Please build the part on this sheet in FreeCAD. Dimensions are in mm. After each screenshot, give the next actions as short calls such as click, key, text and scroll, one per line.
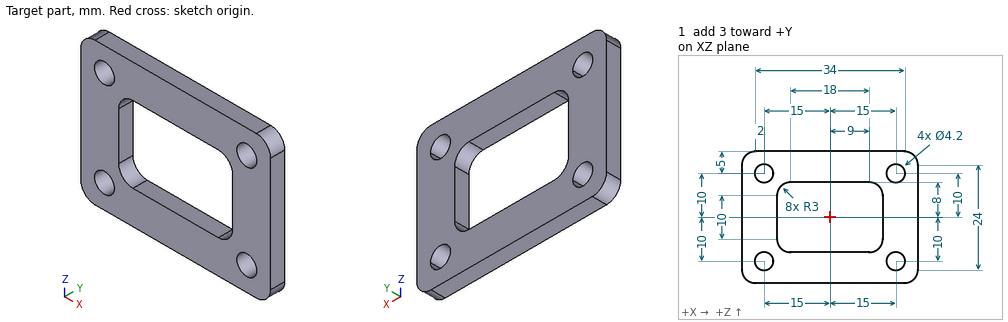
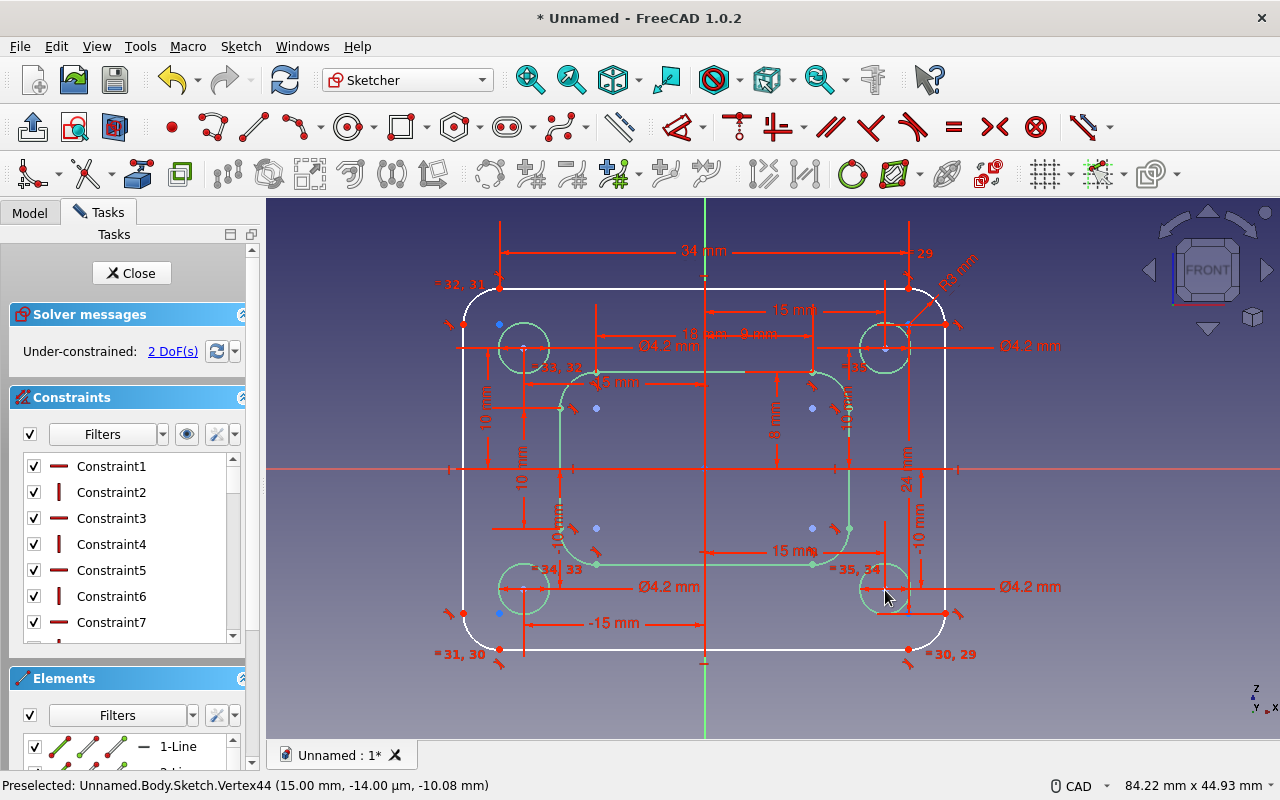
scroll(500, 289, up, 3)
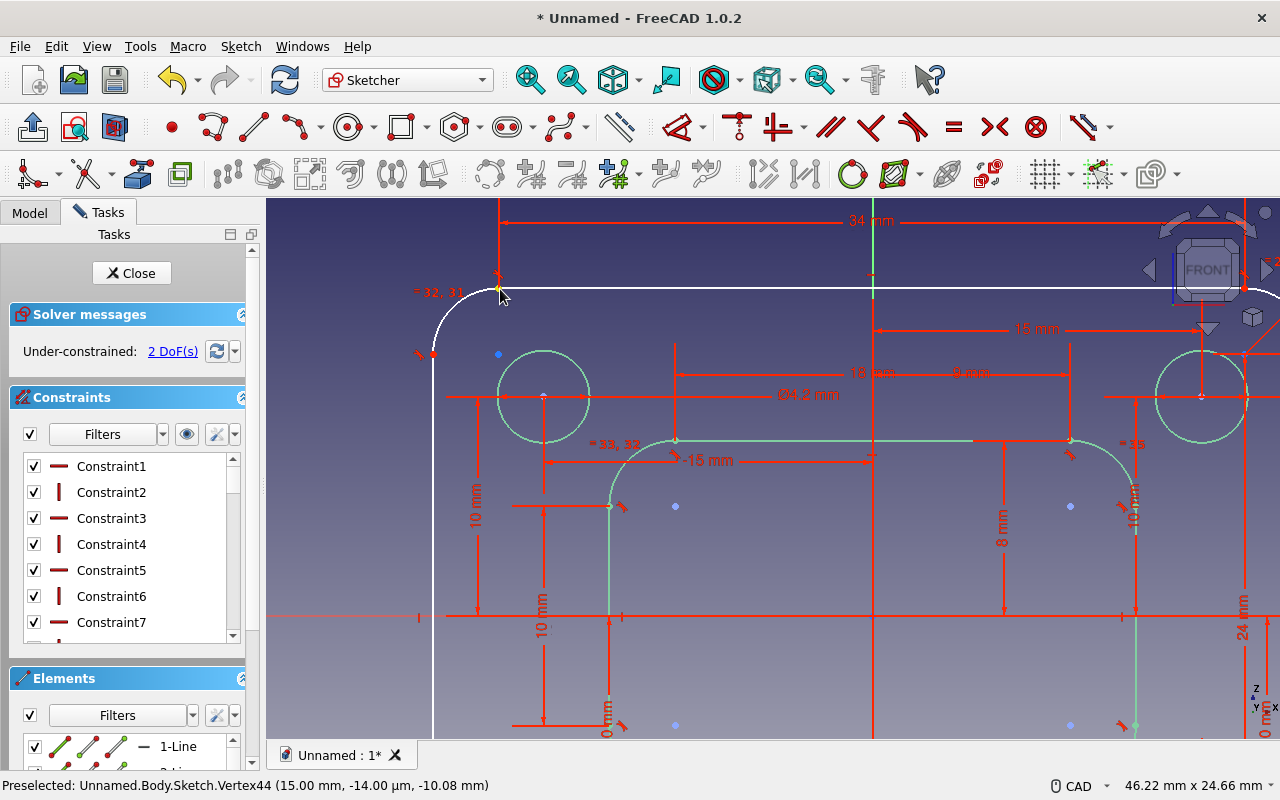
click(499, 288)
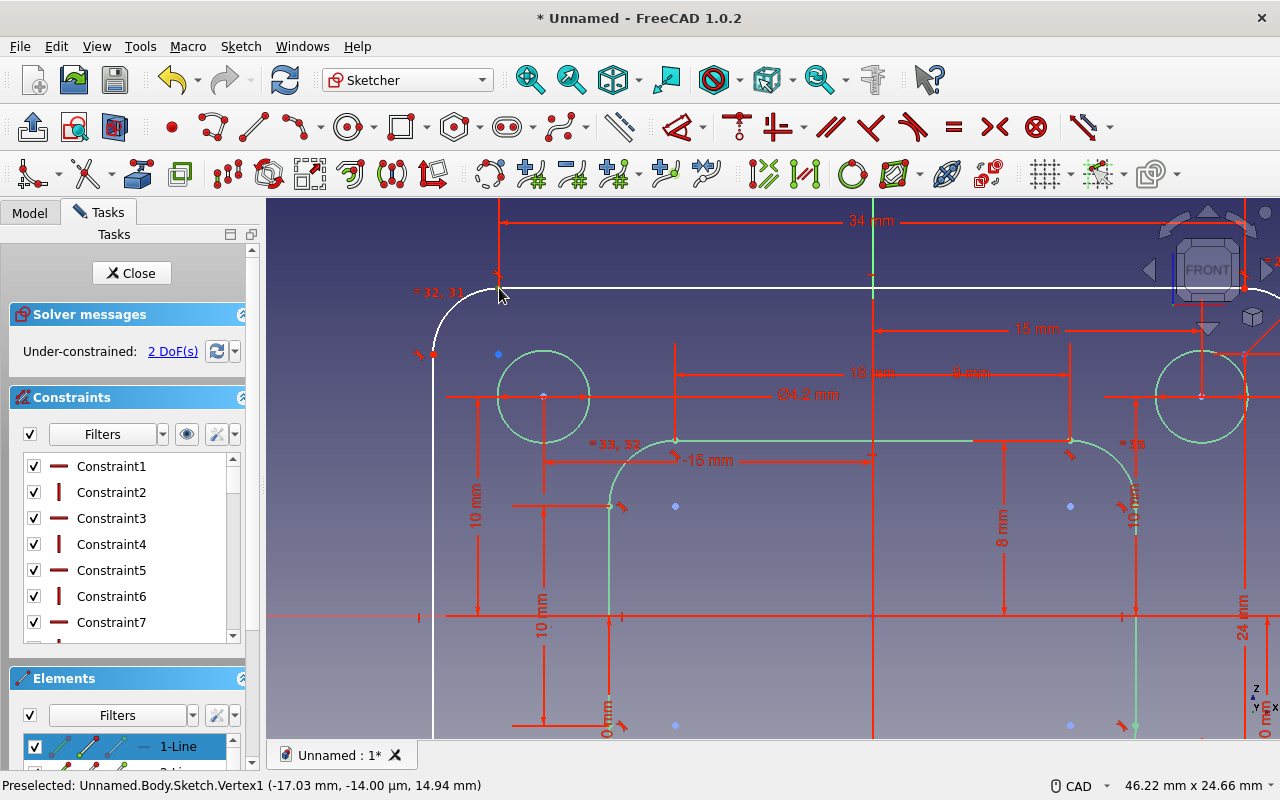
click(544, 397)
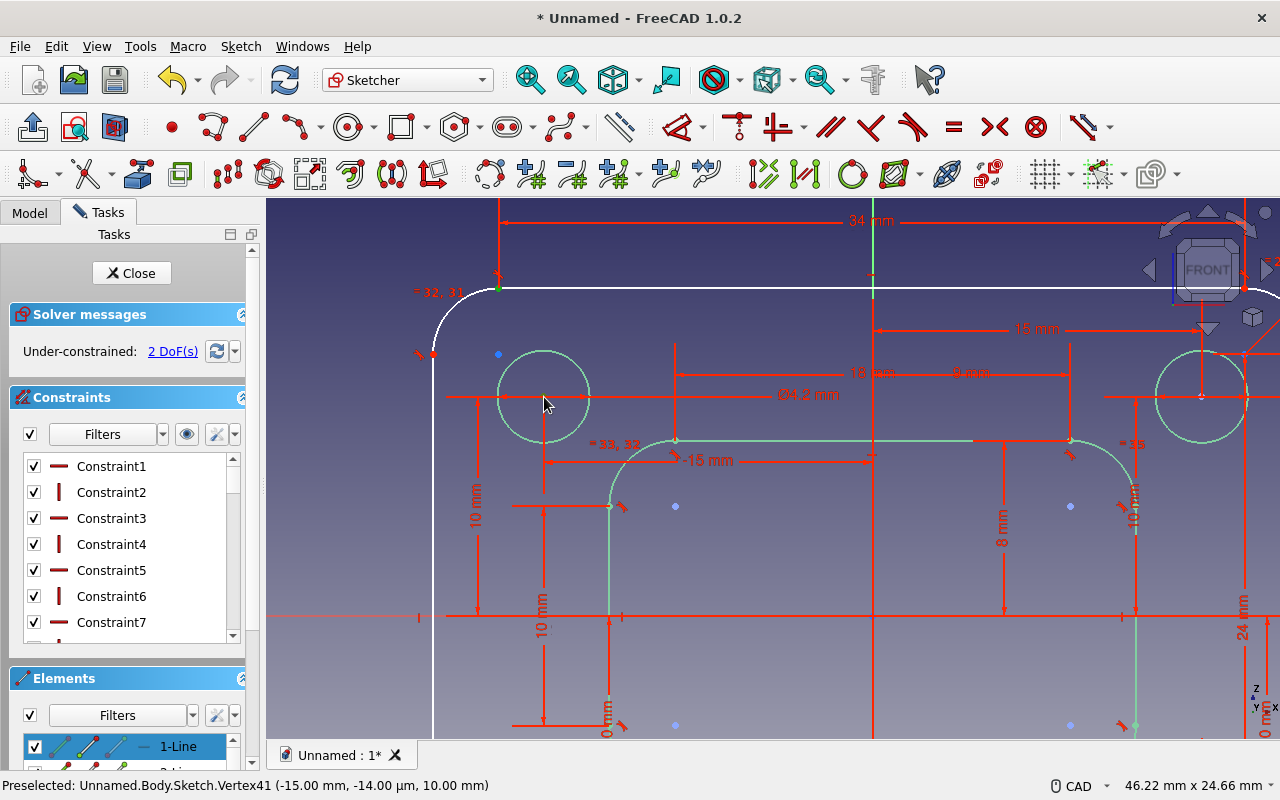
key(l)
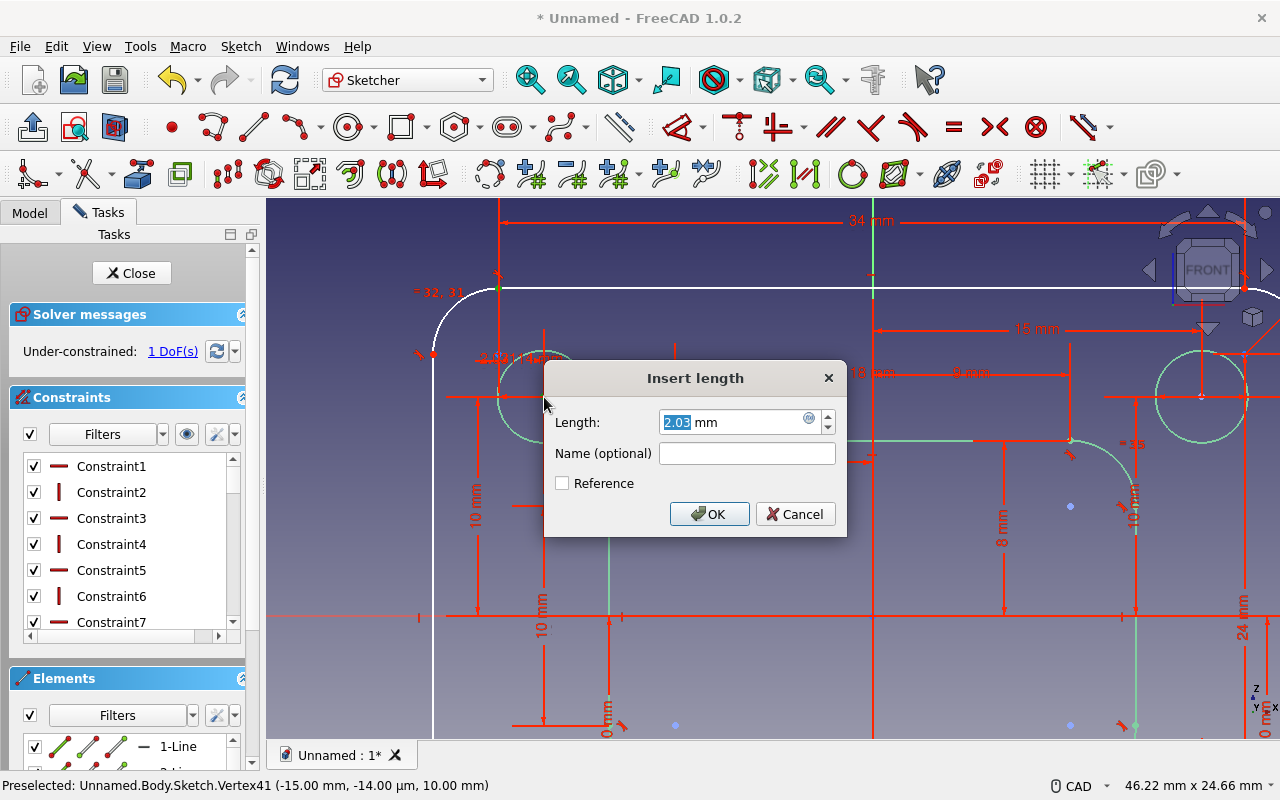
text(2)
key(Return)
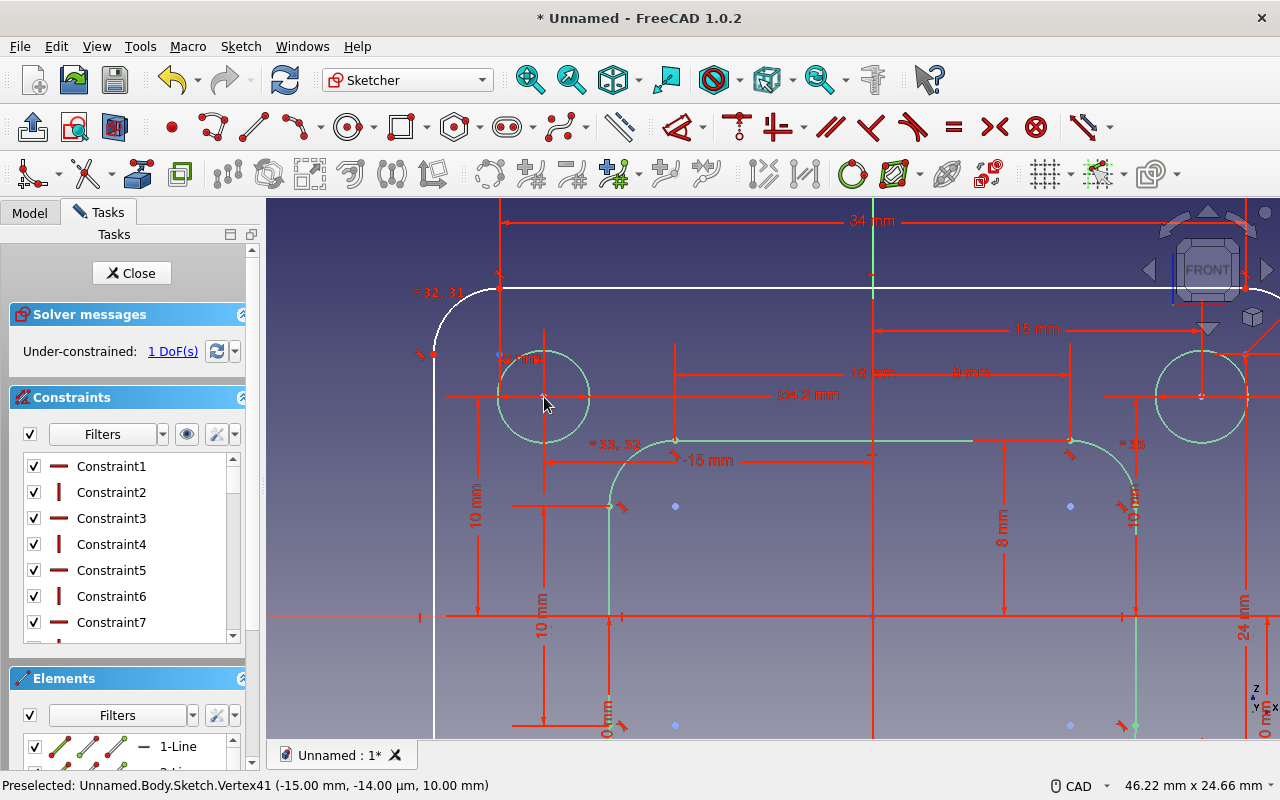
click(500, 288)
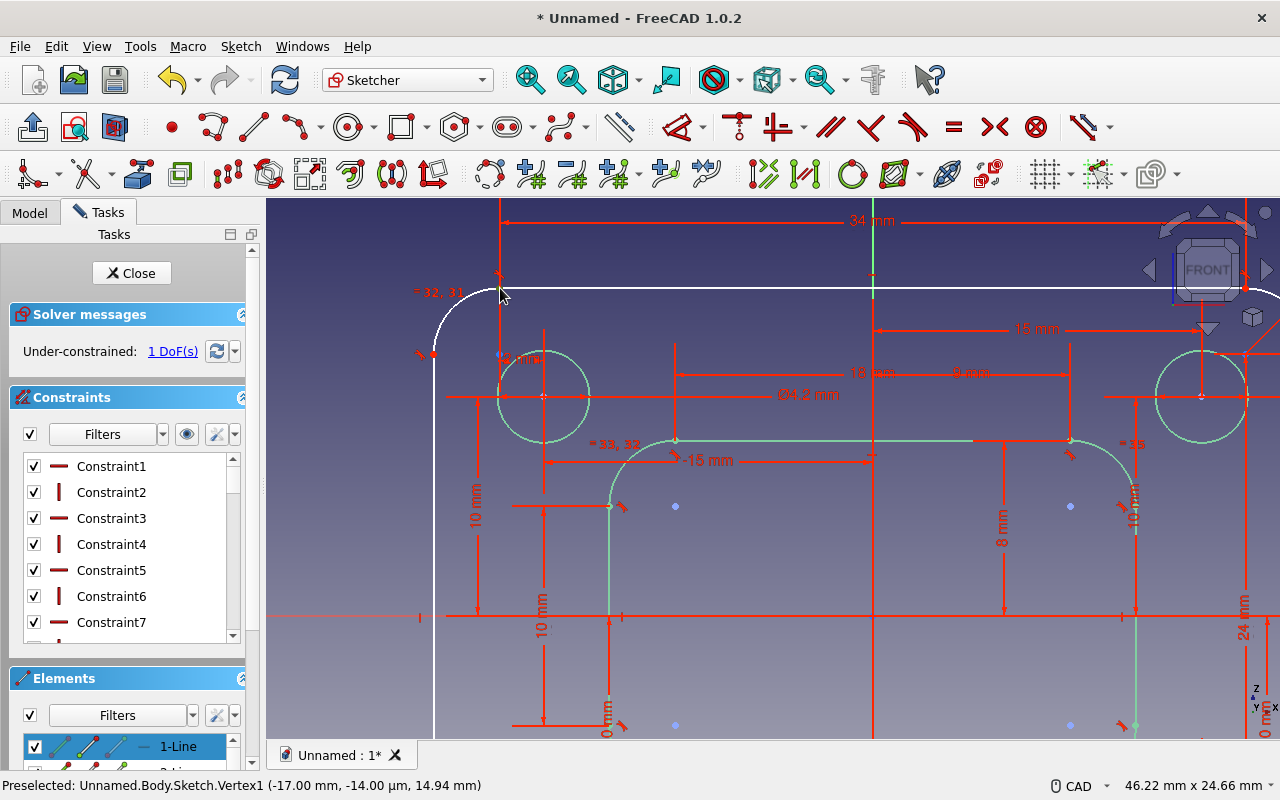
click(544, 397)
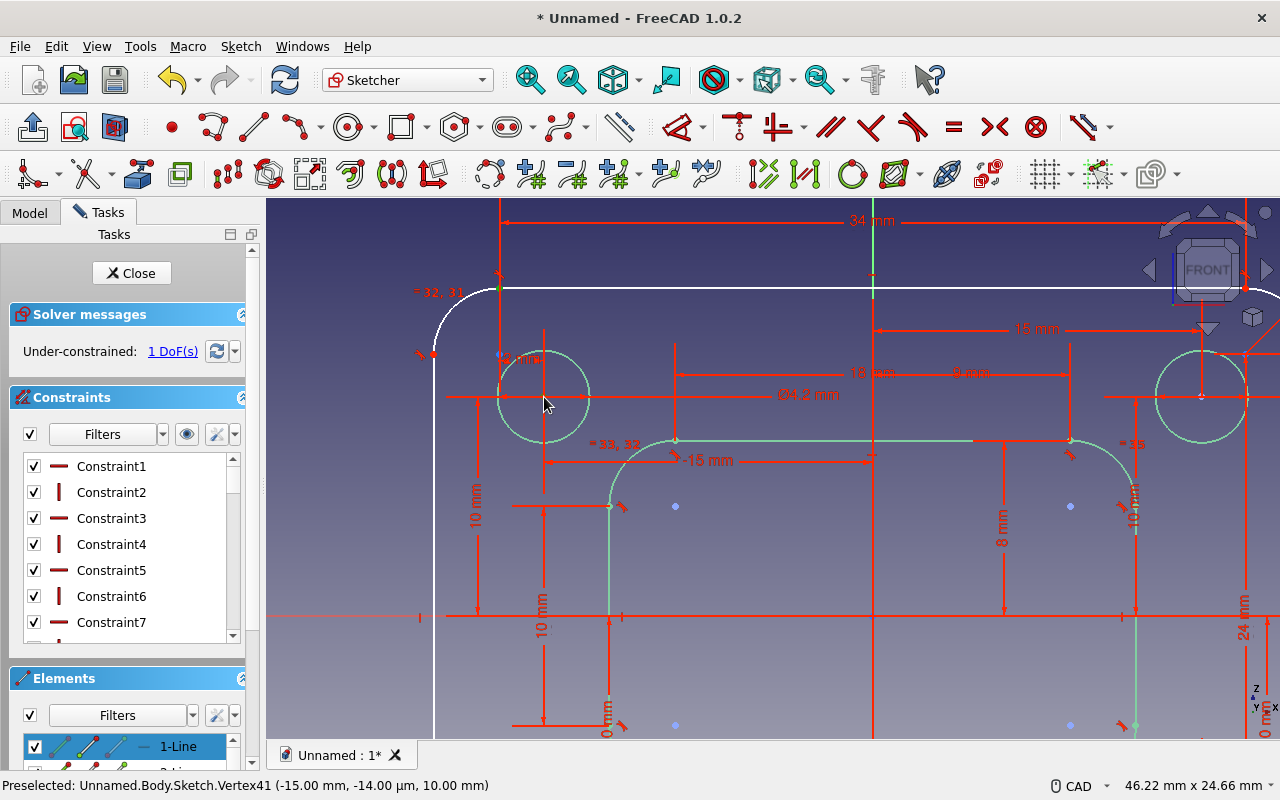
key(i)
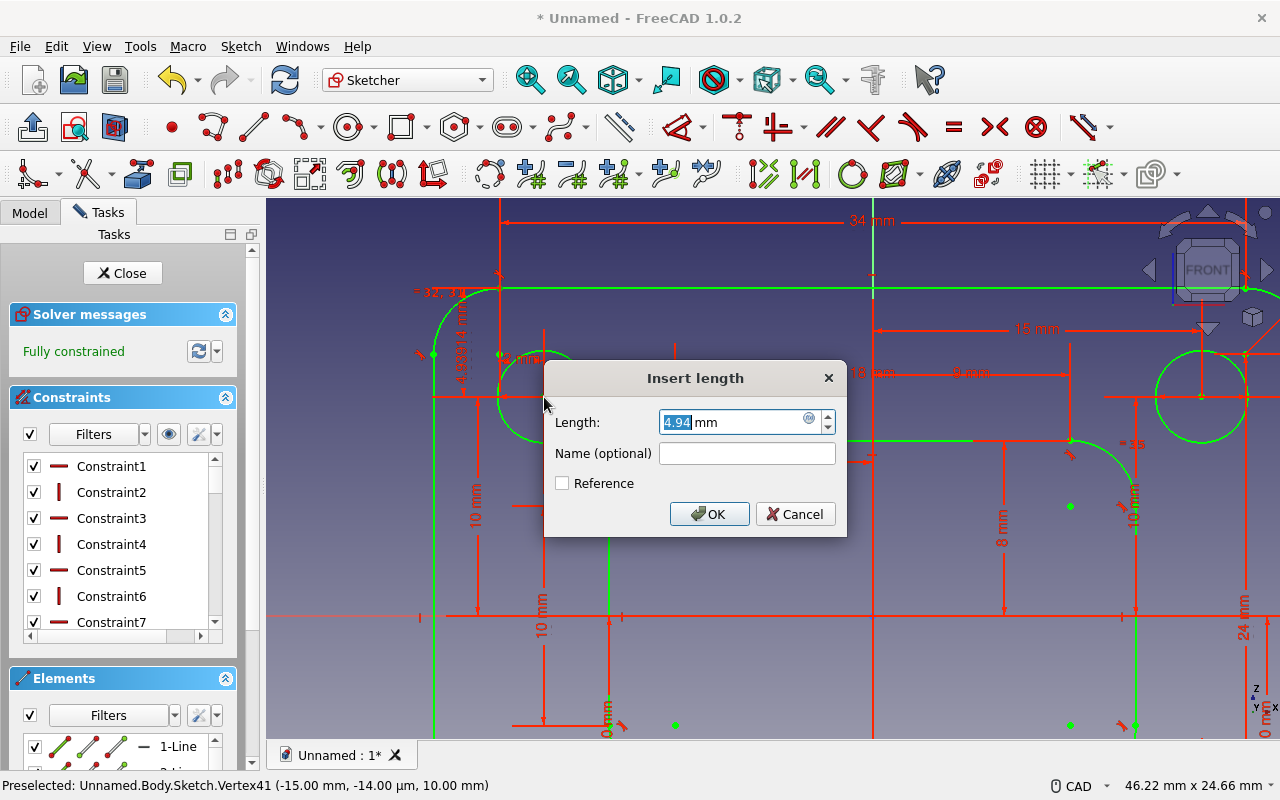
text(5)
key(Return)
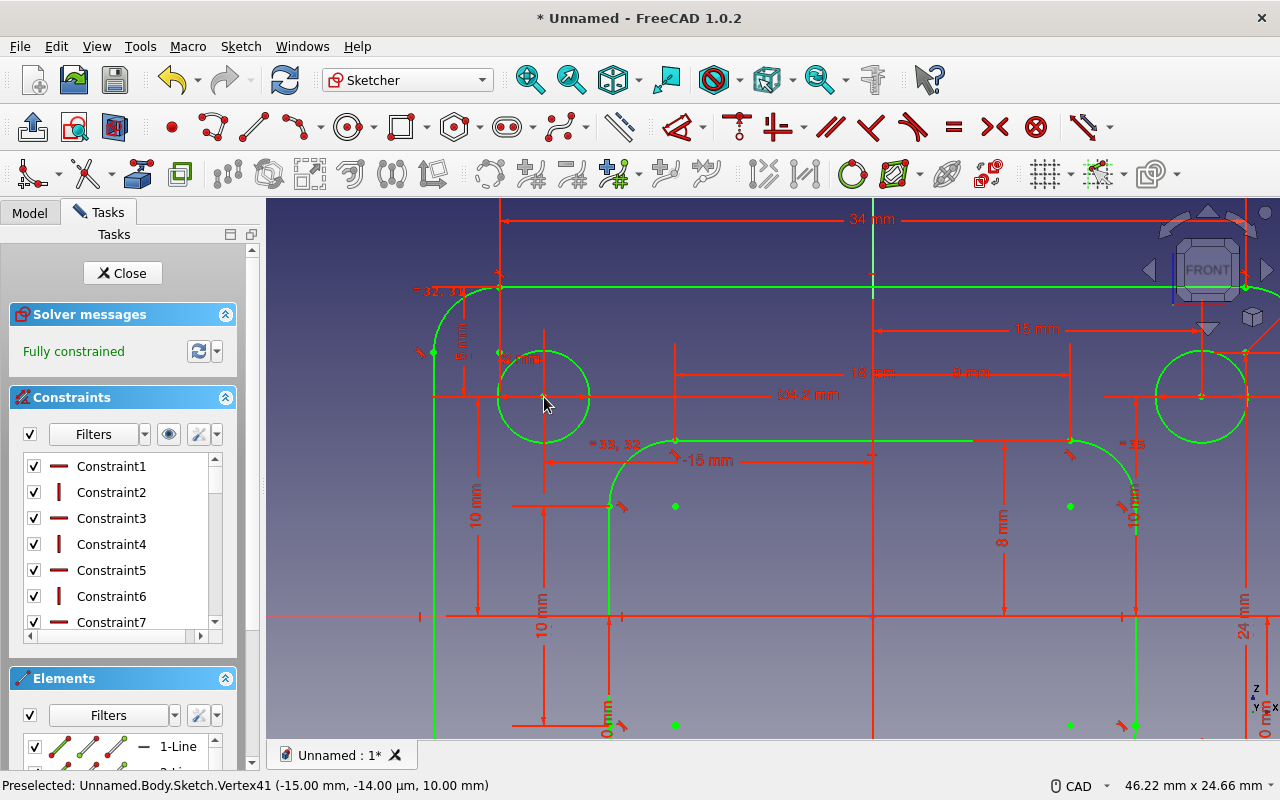
click(123, 273)